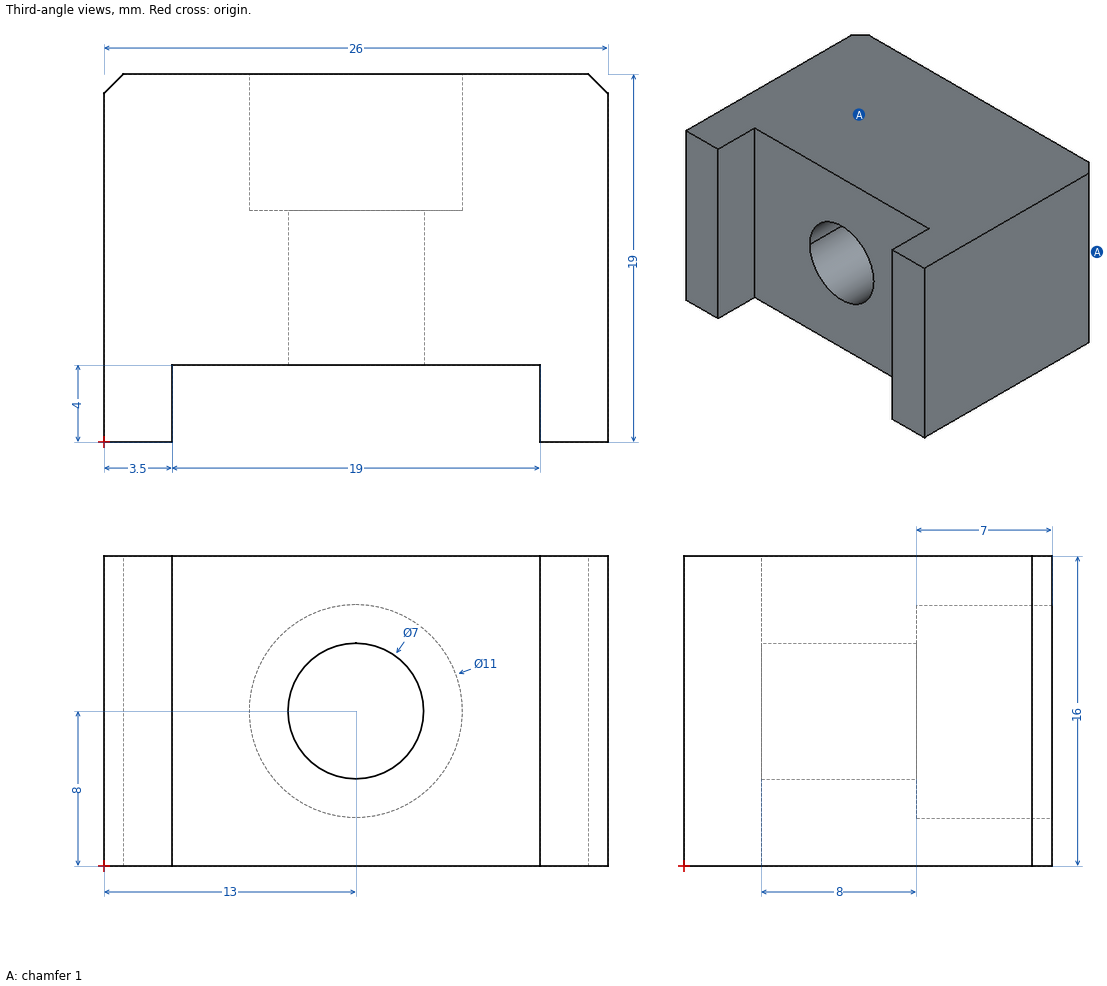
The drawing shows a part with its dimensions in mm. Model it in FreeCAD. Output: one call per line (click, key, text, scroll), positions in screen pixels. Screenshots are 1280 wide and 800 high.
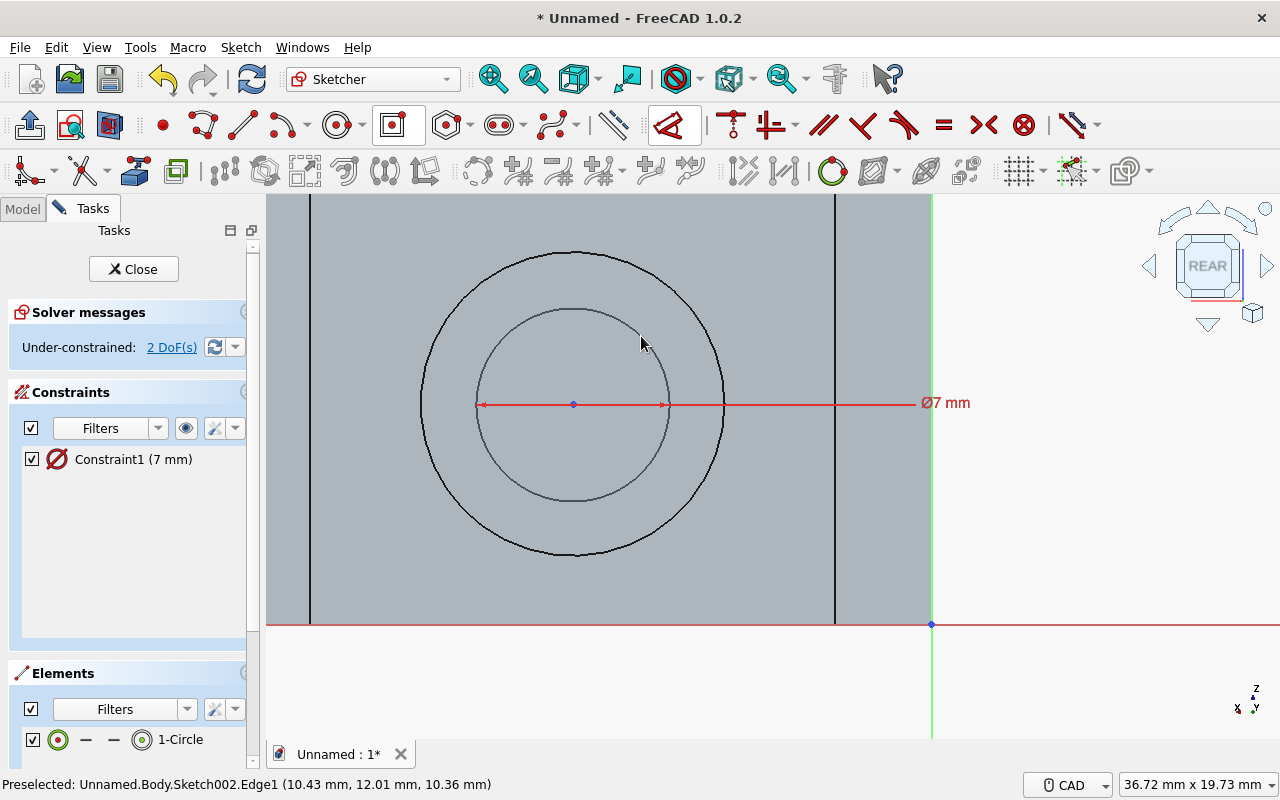
click(573, 405)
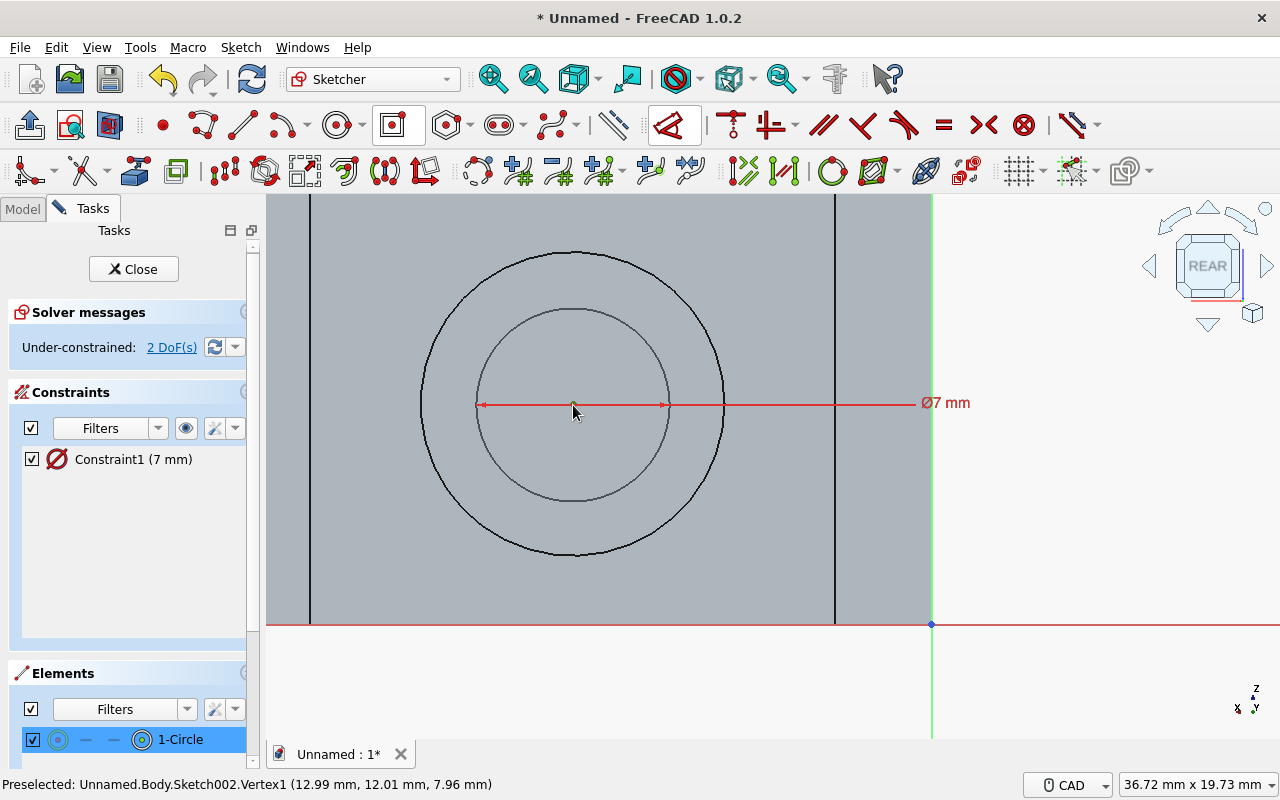
click(696, 126)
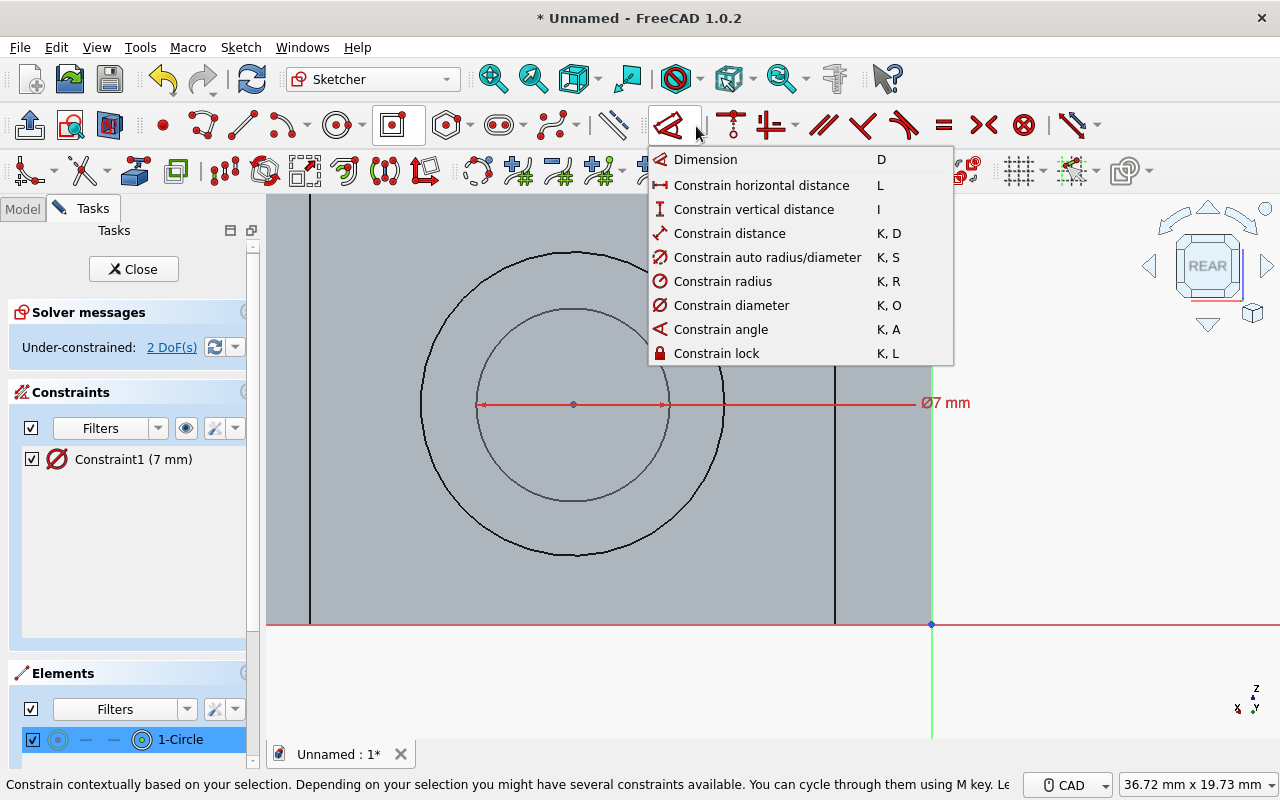
click(801, 209)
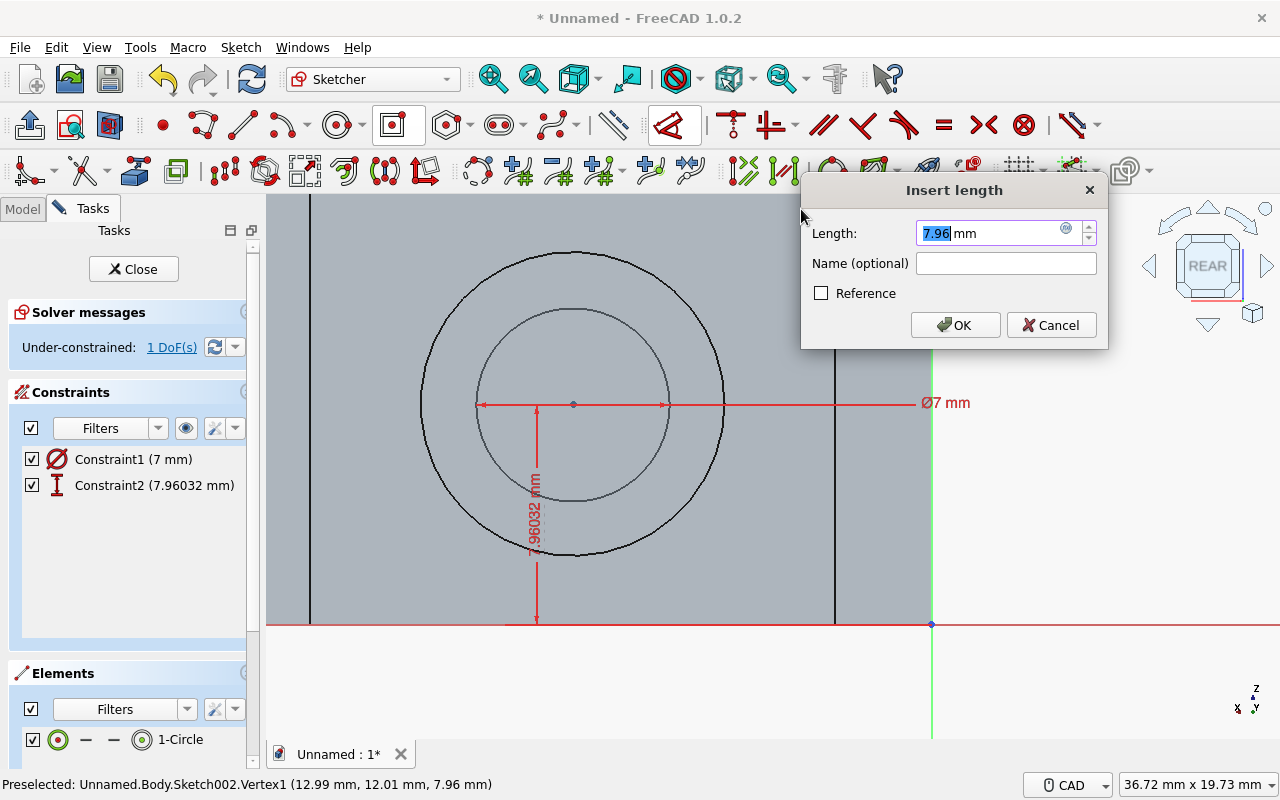
text(8)
key(Return)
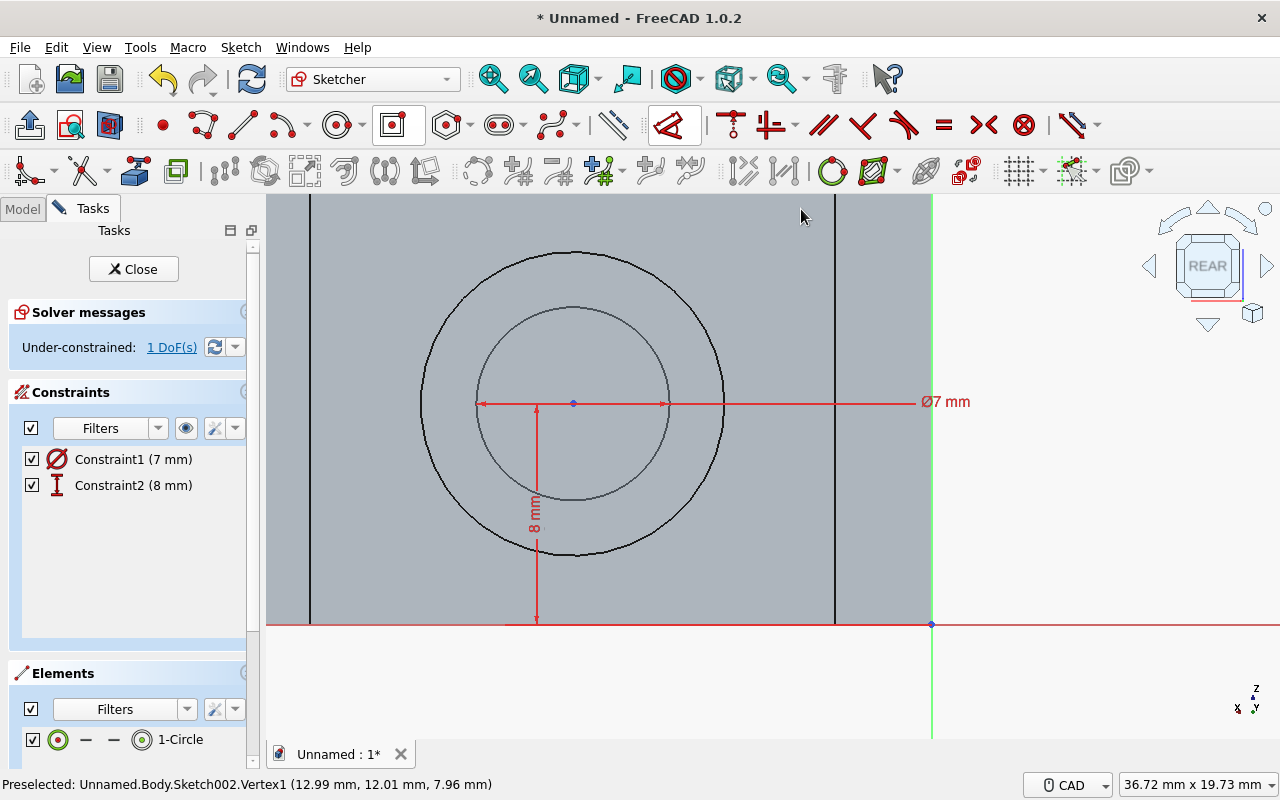
click(573, 404)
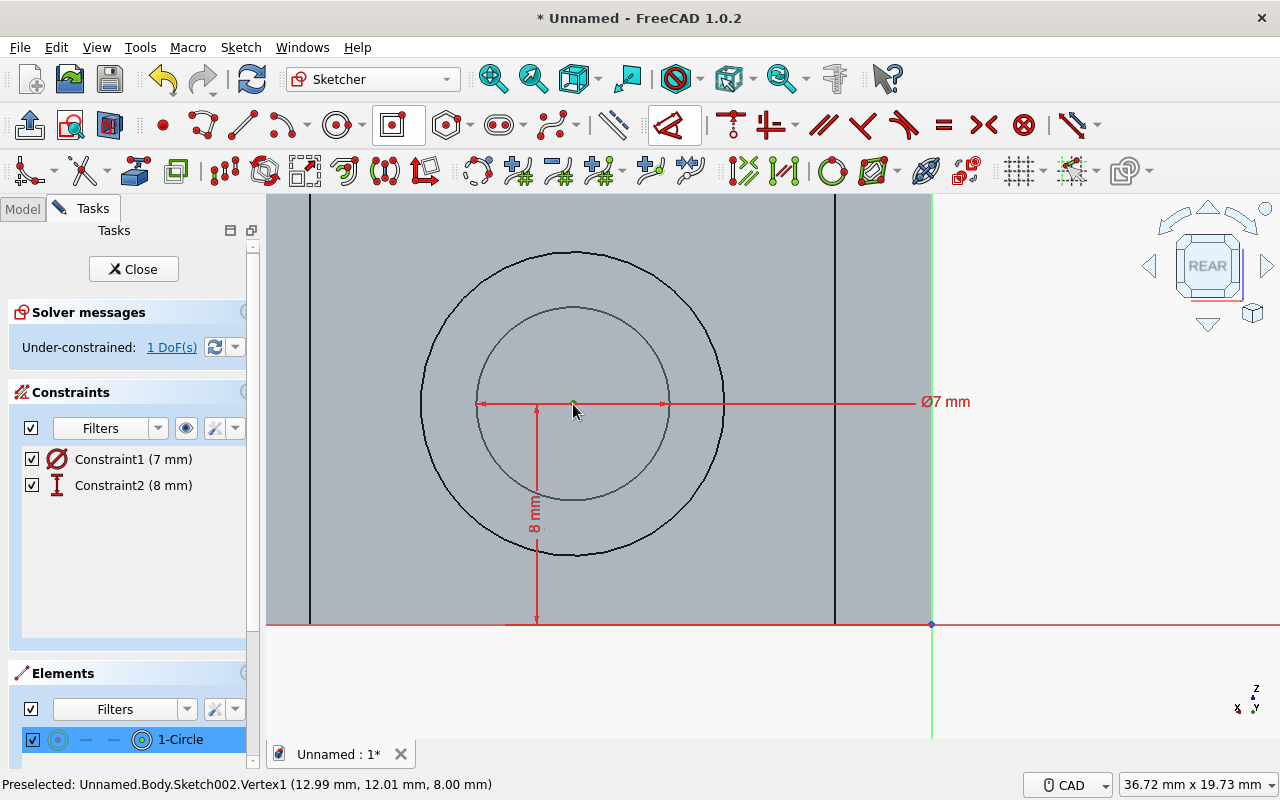
key(l)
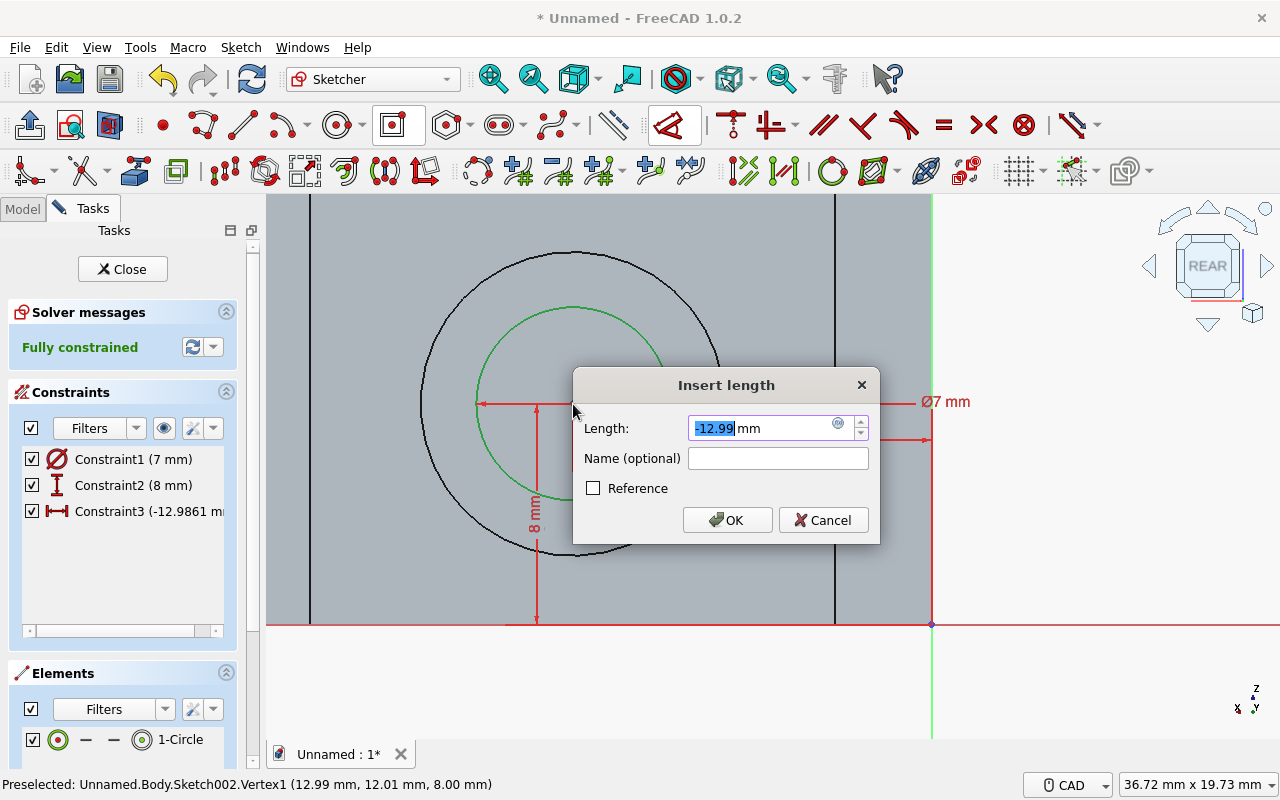
text(-13)
key(Return)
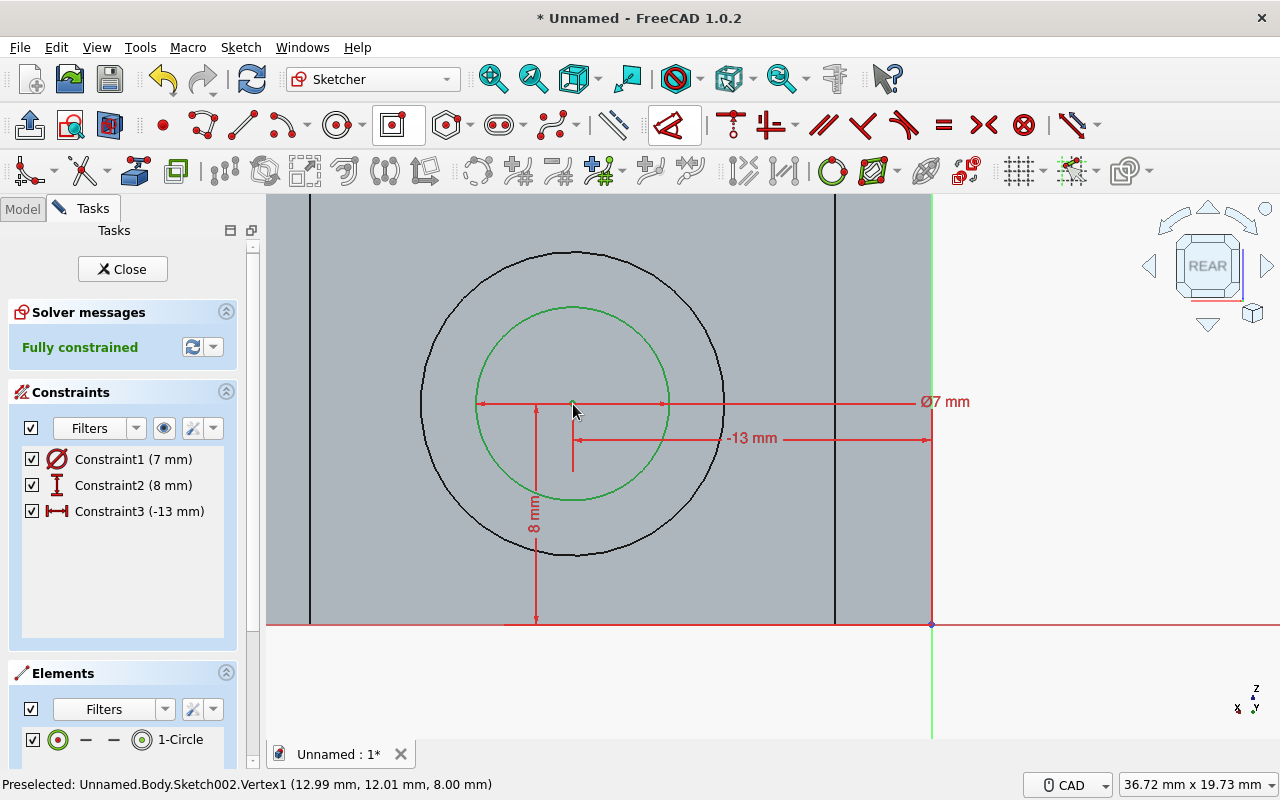
click(123, 269)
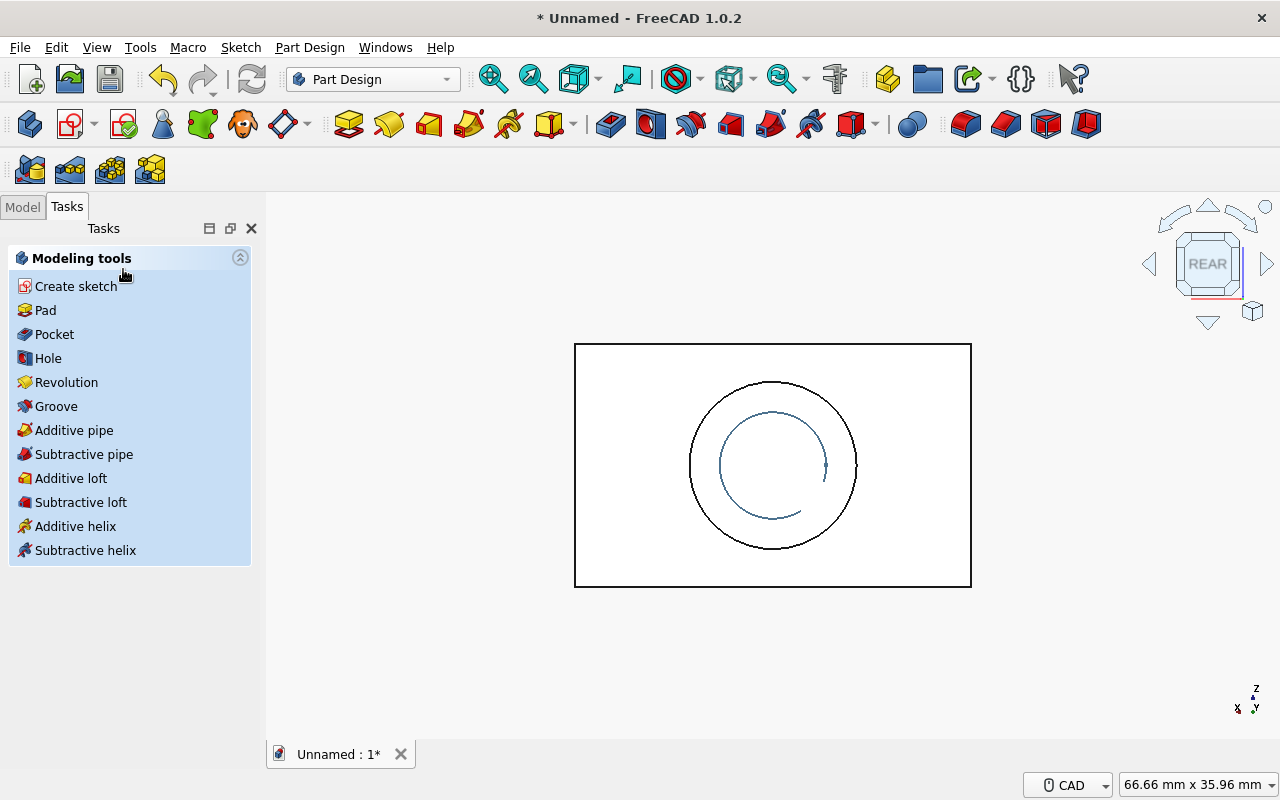
click(612, 124)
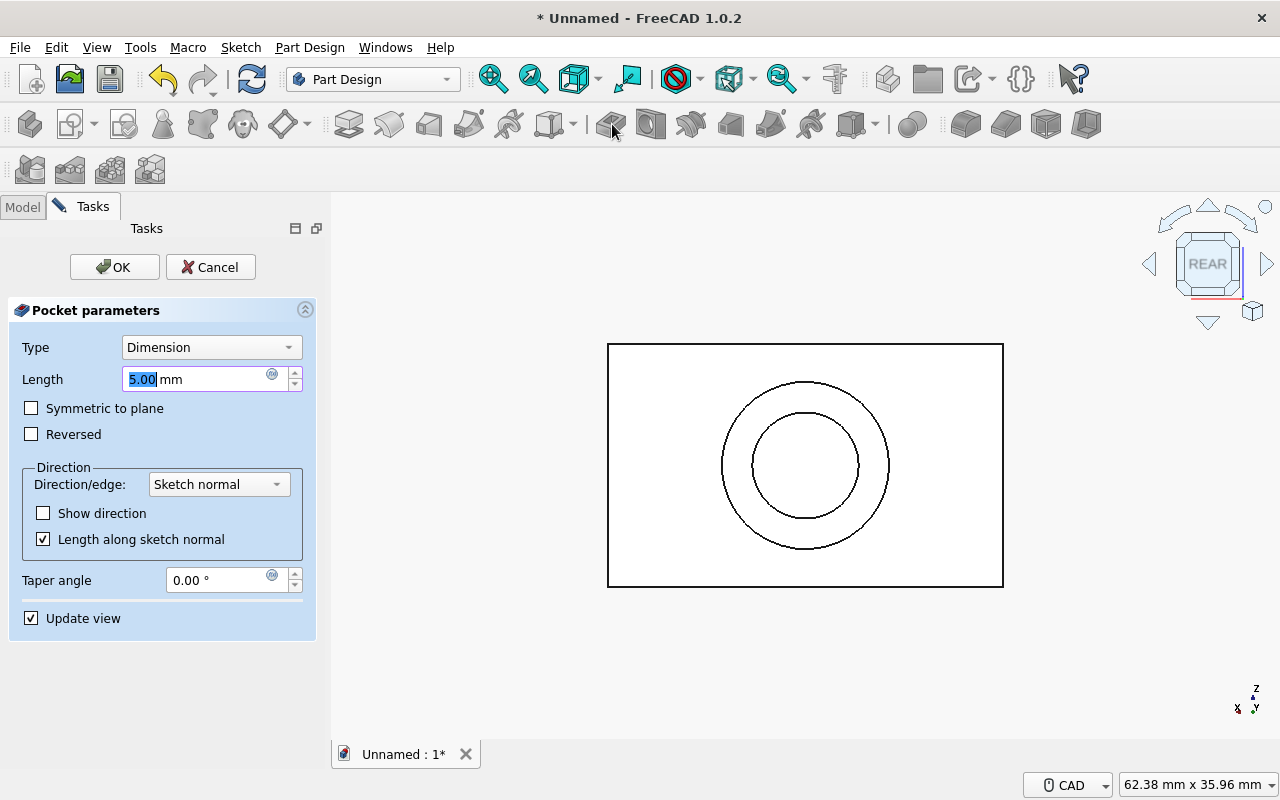
text(8)
key(Tab)